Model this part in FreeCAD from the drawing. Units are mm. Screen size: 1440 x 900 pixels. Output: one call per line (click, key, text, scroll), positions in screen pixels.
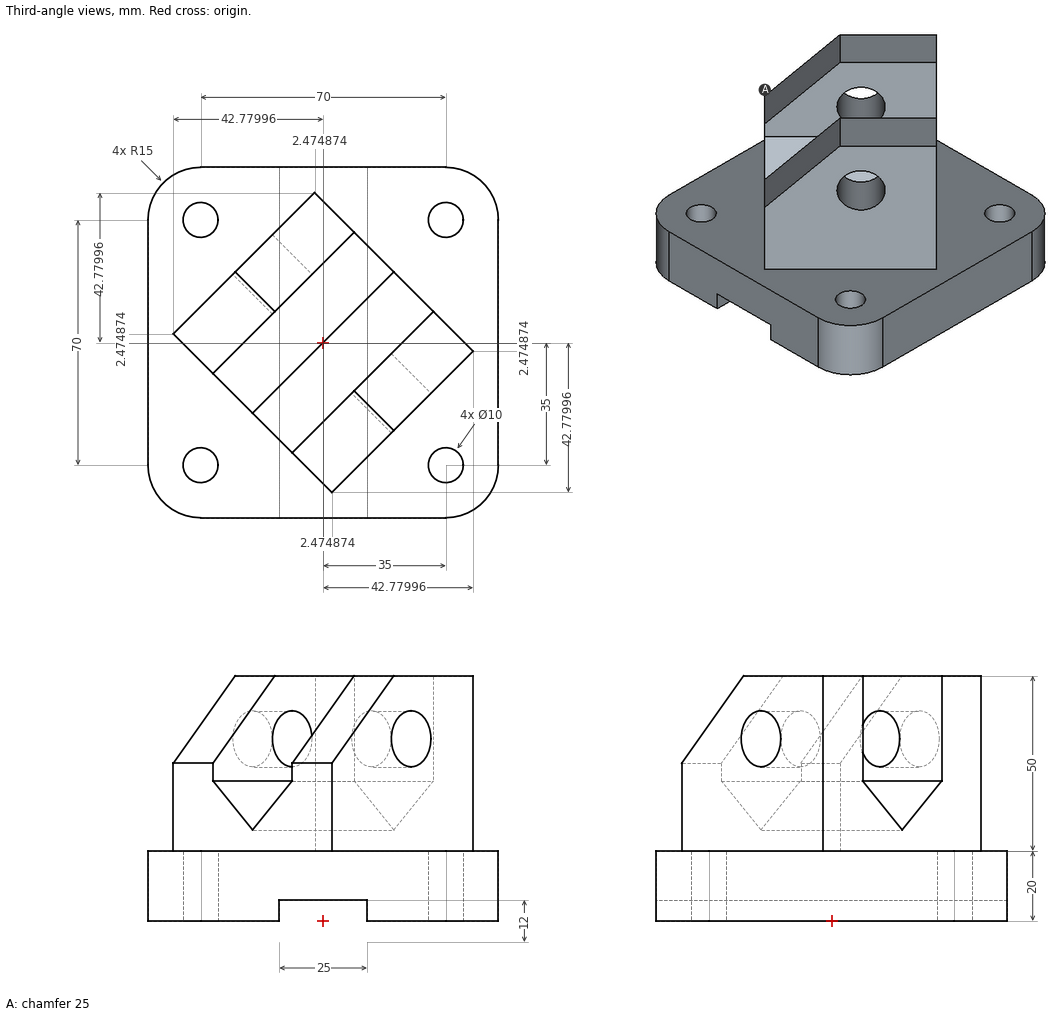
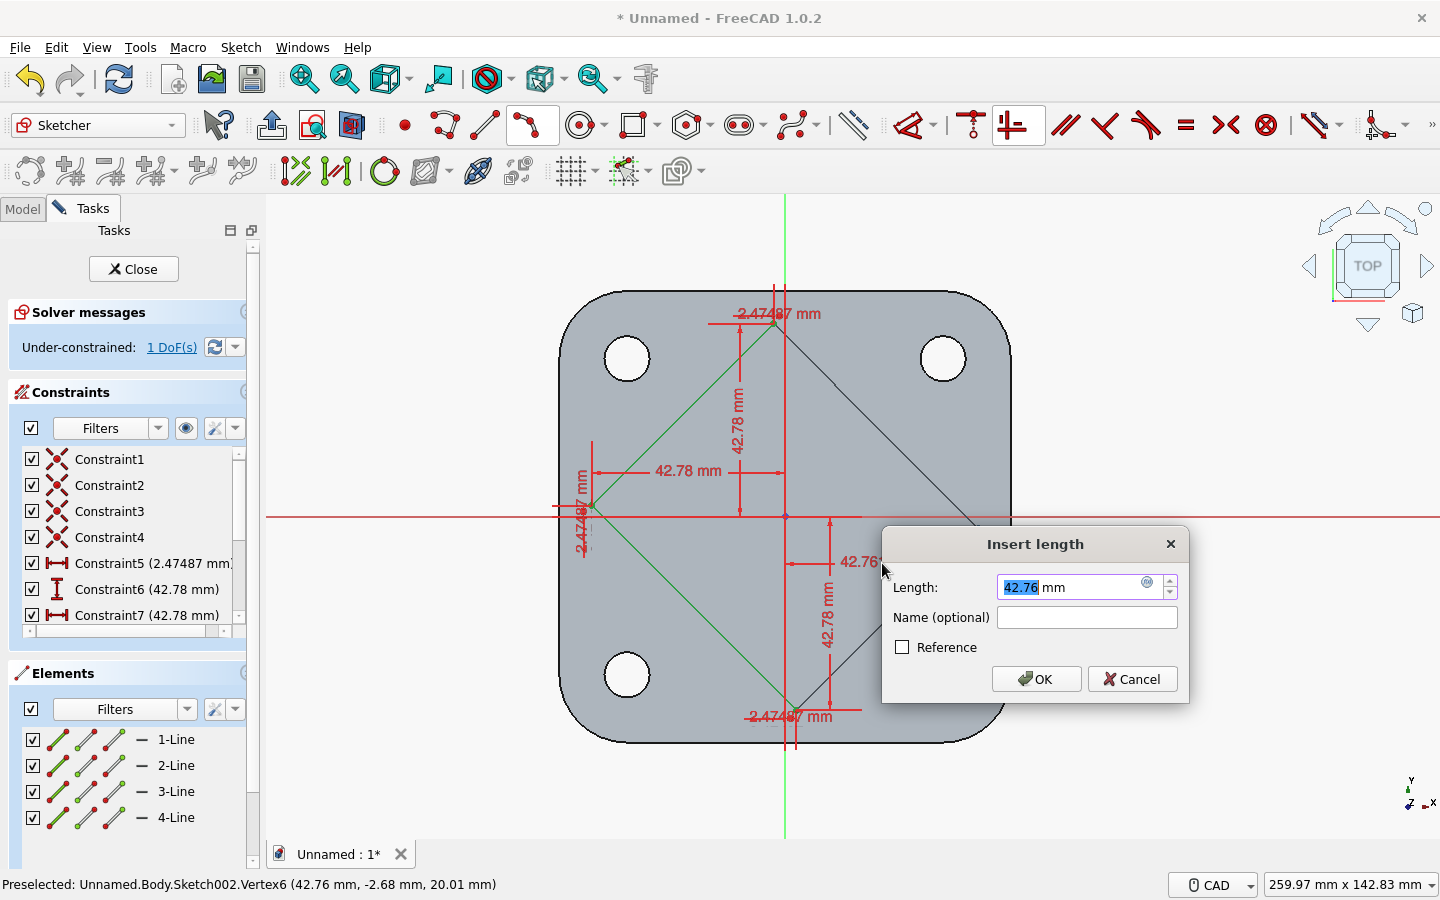
text(42.77996)
key(Return)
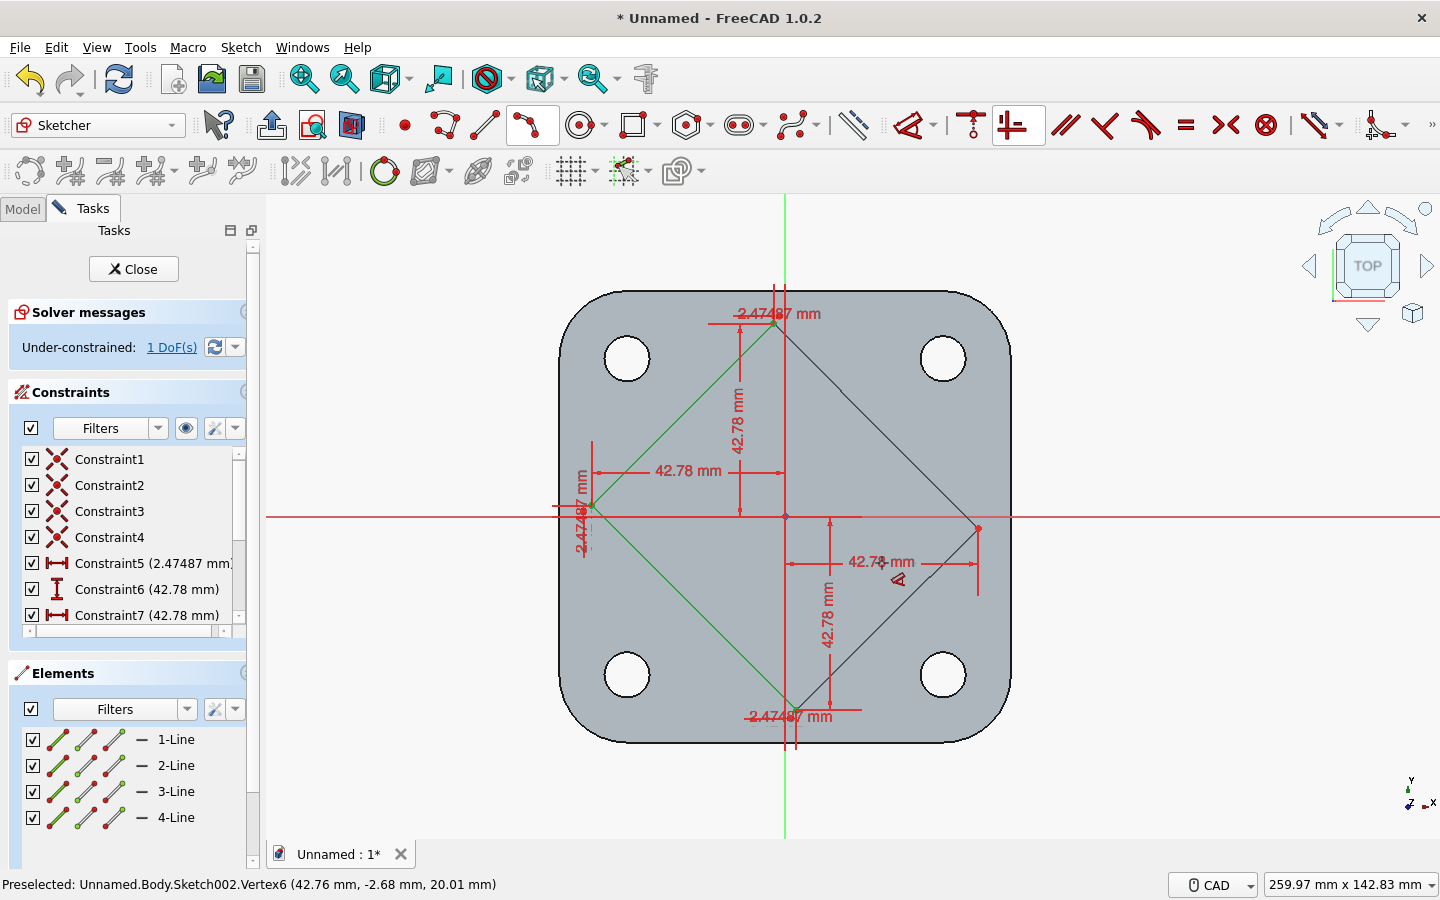
scroll(978, 529, up, 7)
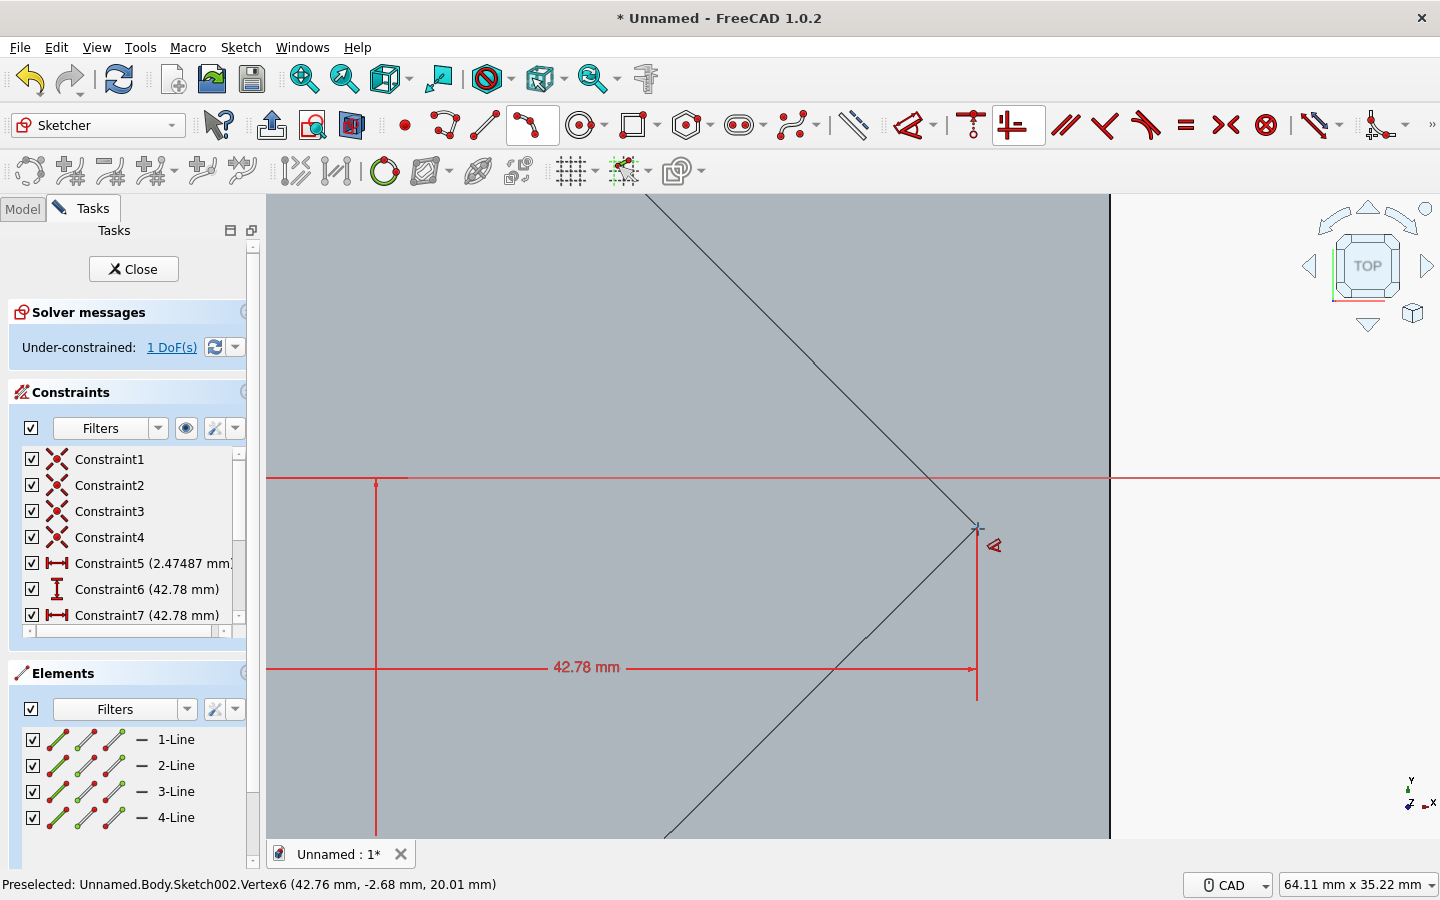
click(977, 527)
click(1011, 503)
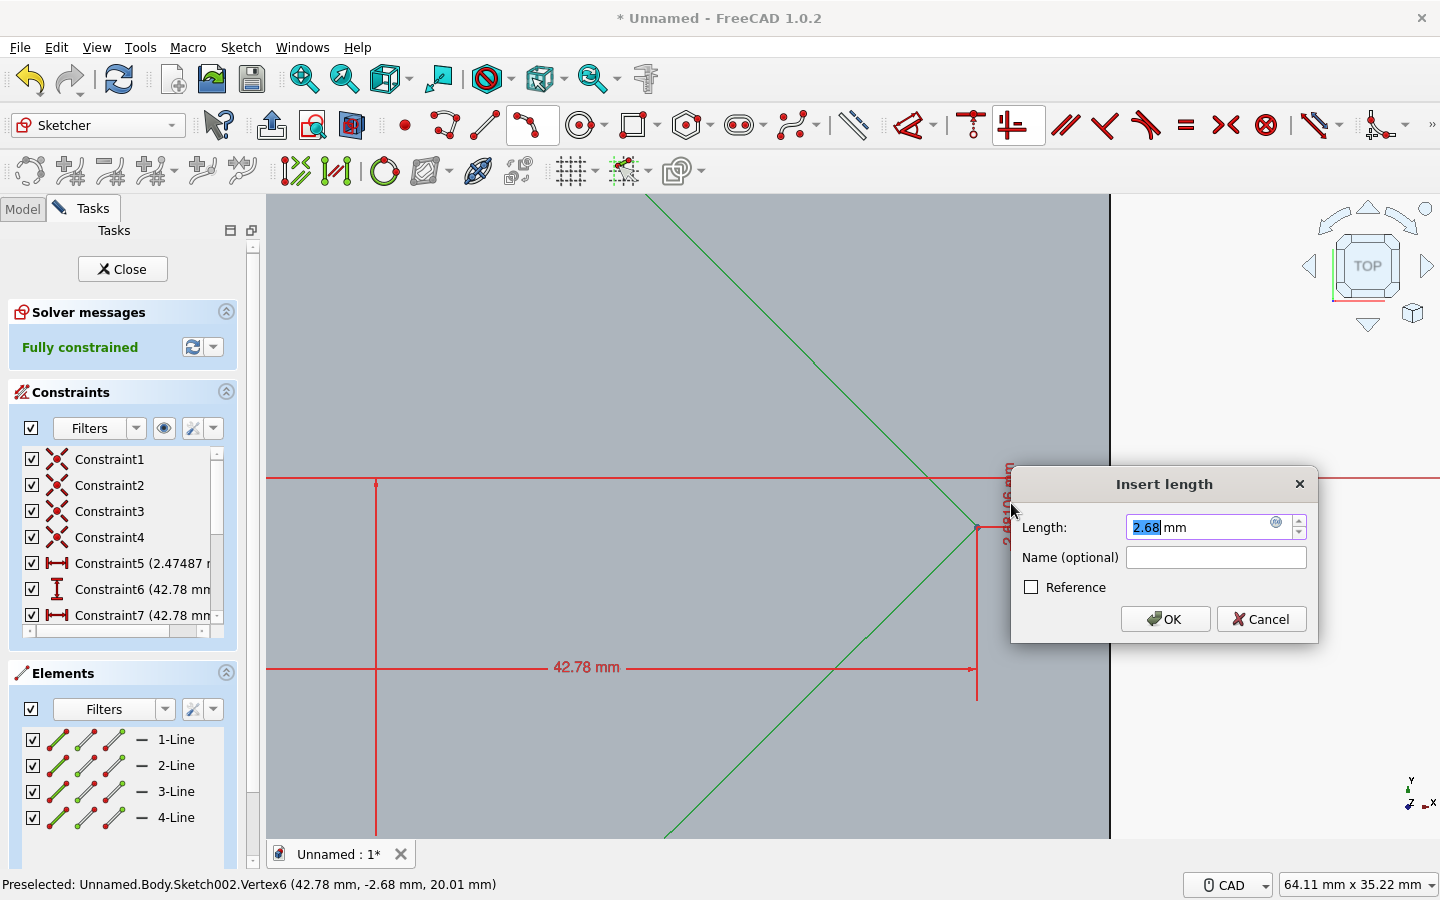
text(2.474874)
key(Return)
key(Escape)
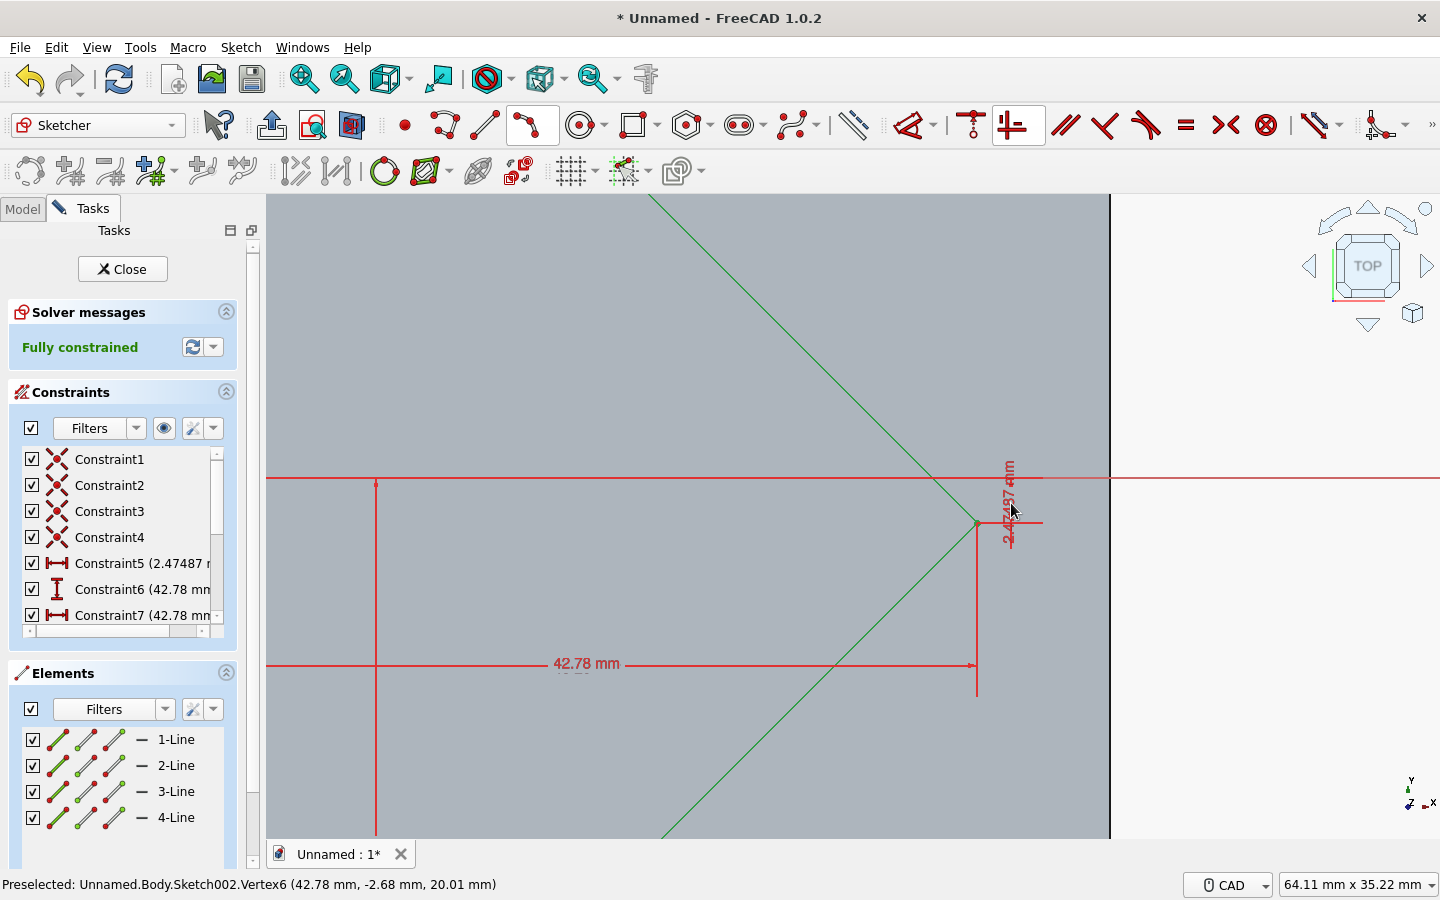
click(123, 269)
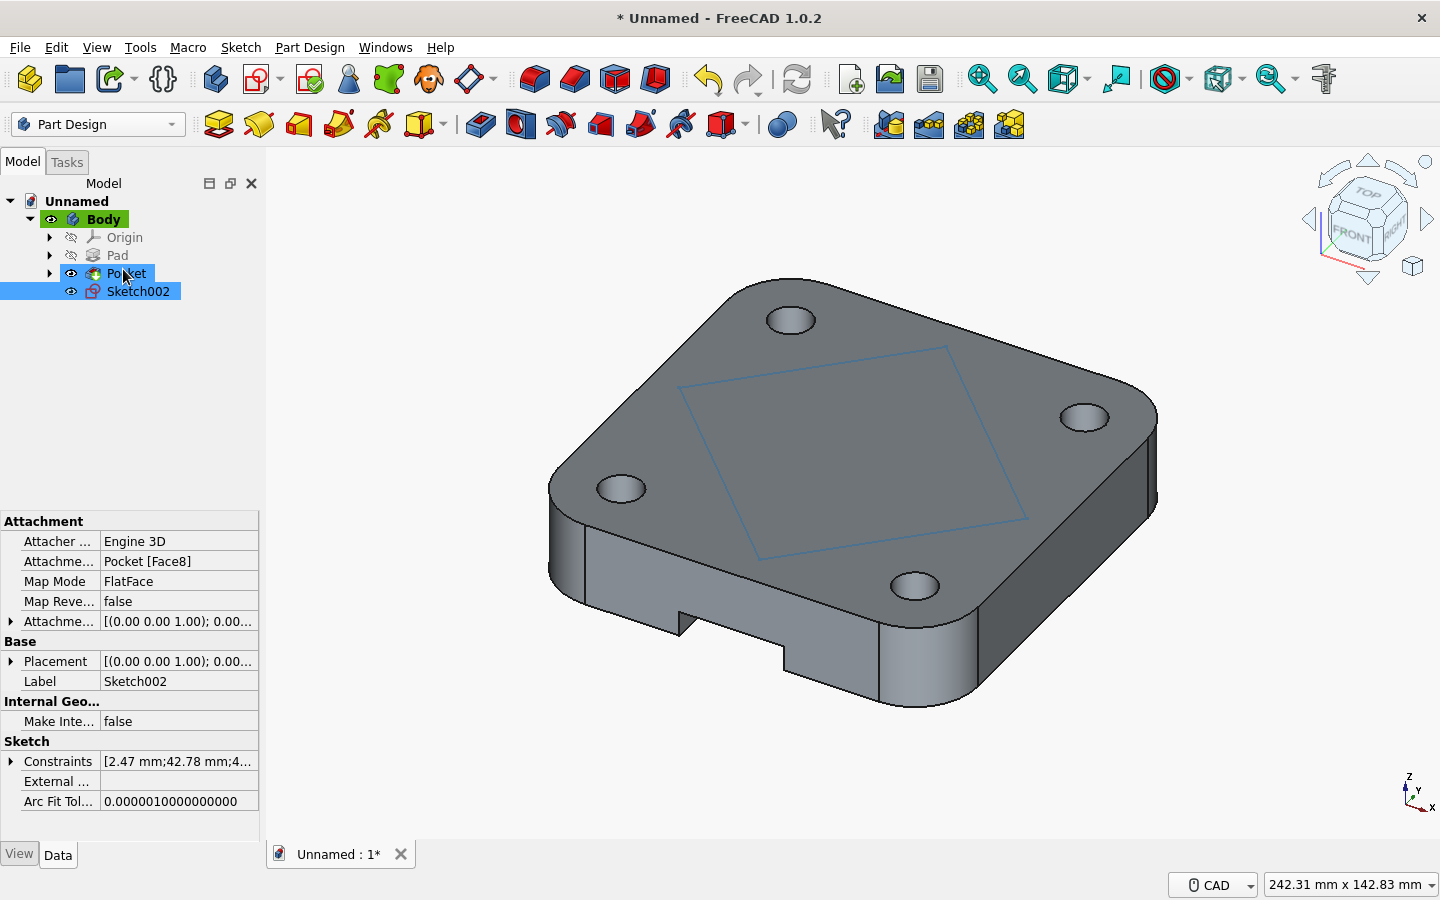
click(220, 124)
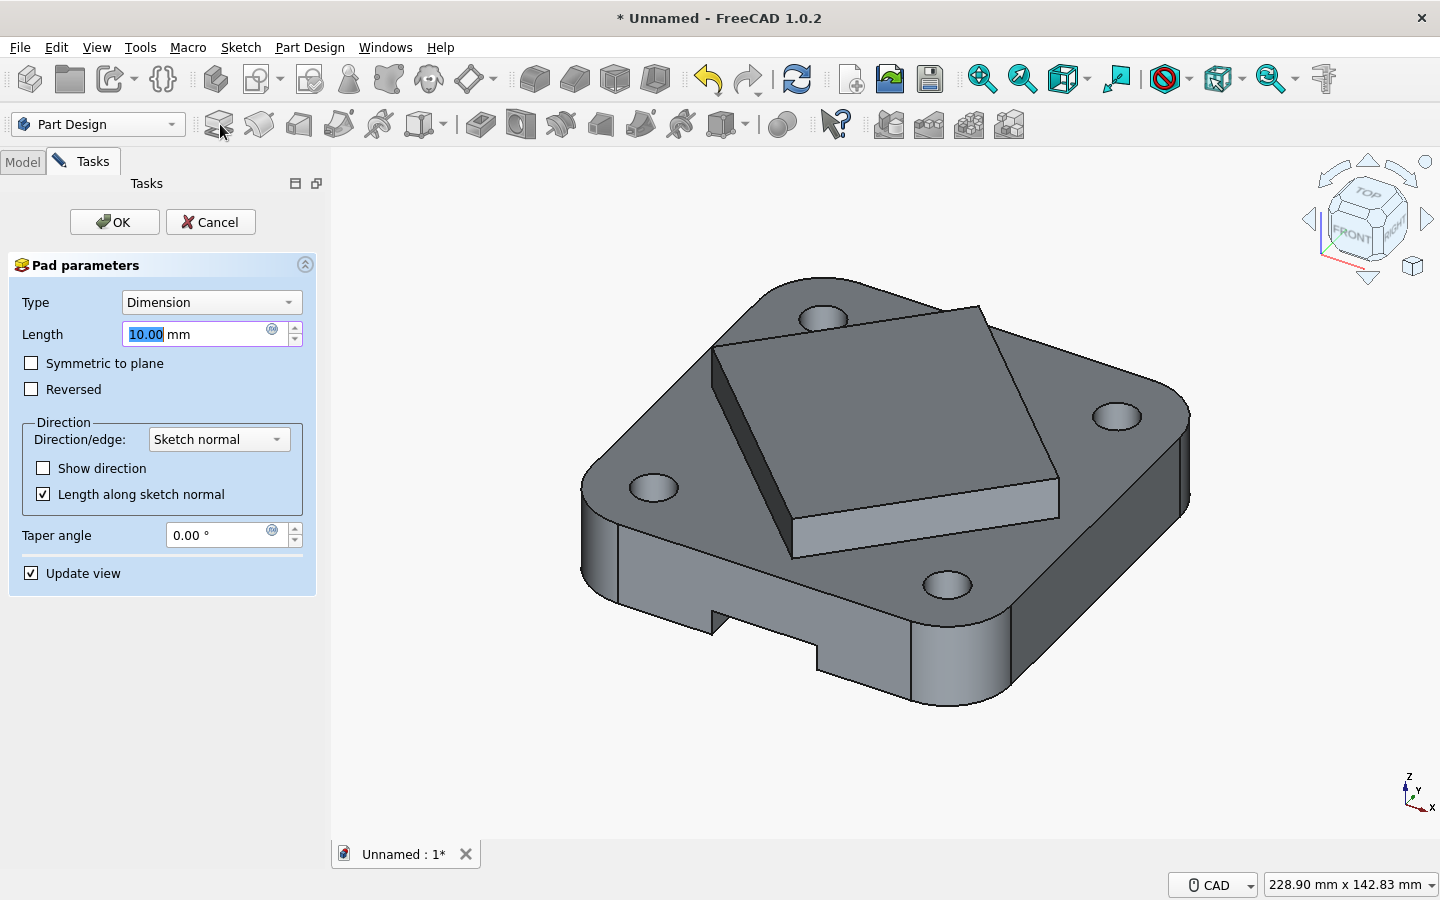
text(50)
key(Tab)